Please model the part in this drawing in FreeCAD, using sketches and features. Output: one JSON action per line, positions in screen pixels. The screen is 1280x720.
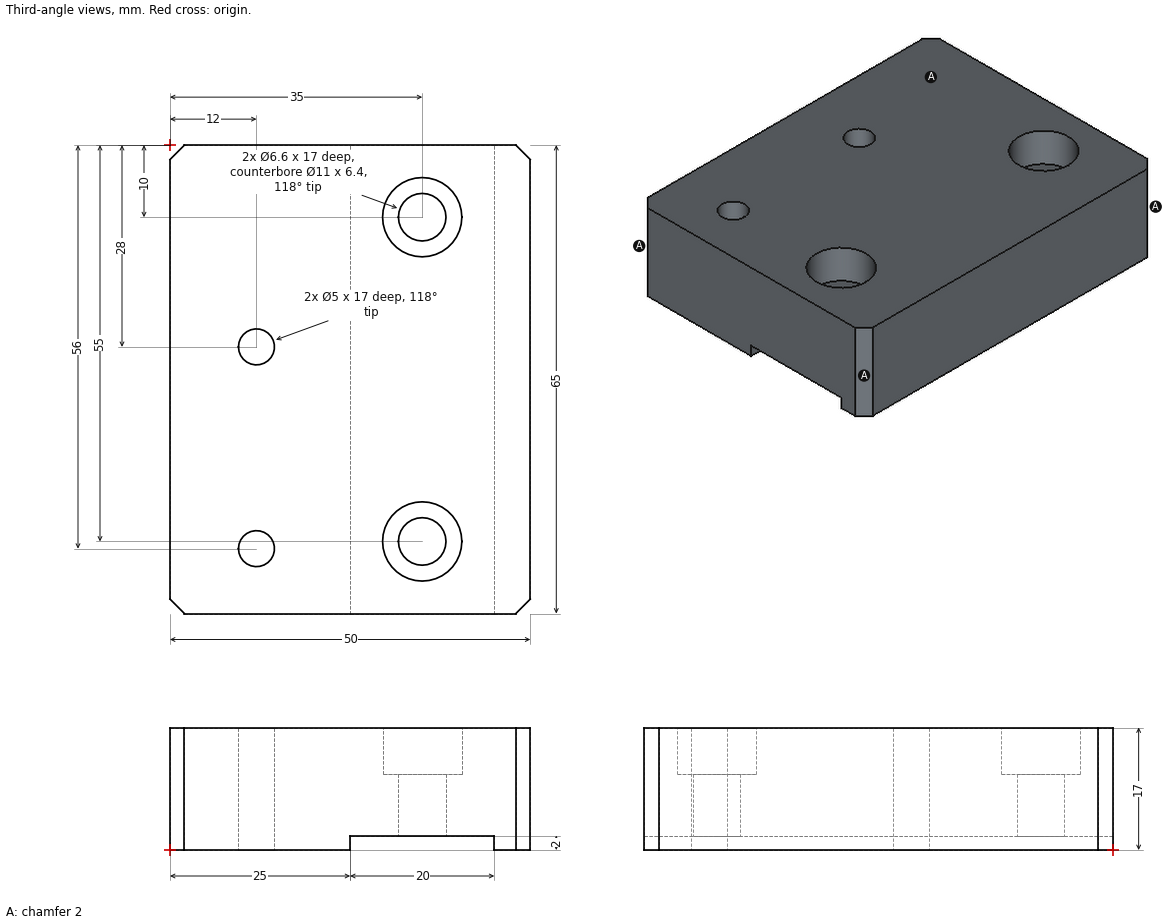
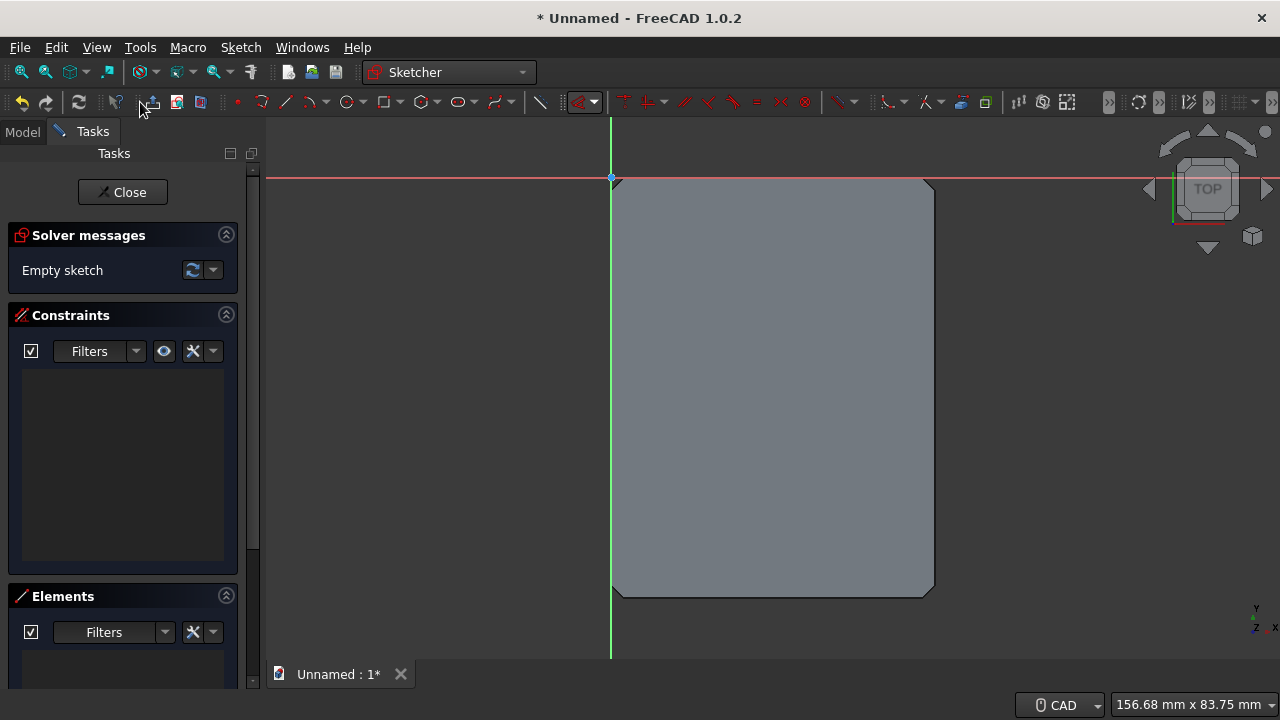
{"action": "left_click", "coordinate": [348, 102]}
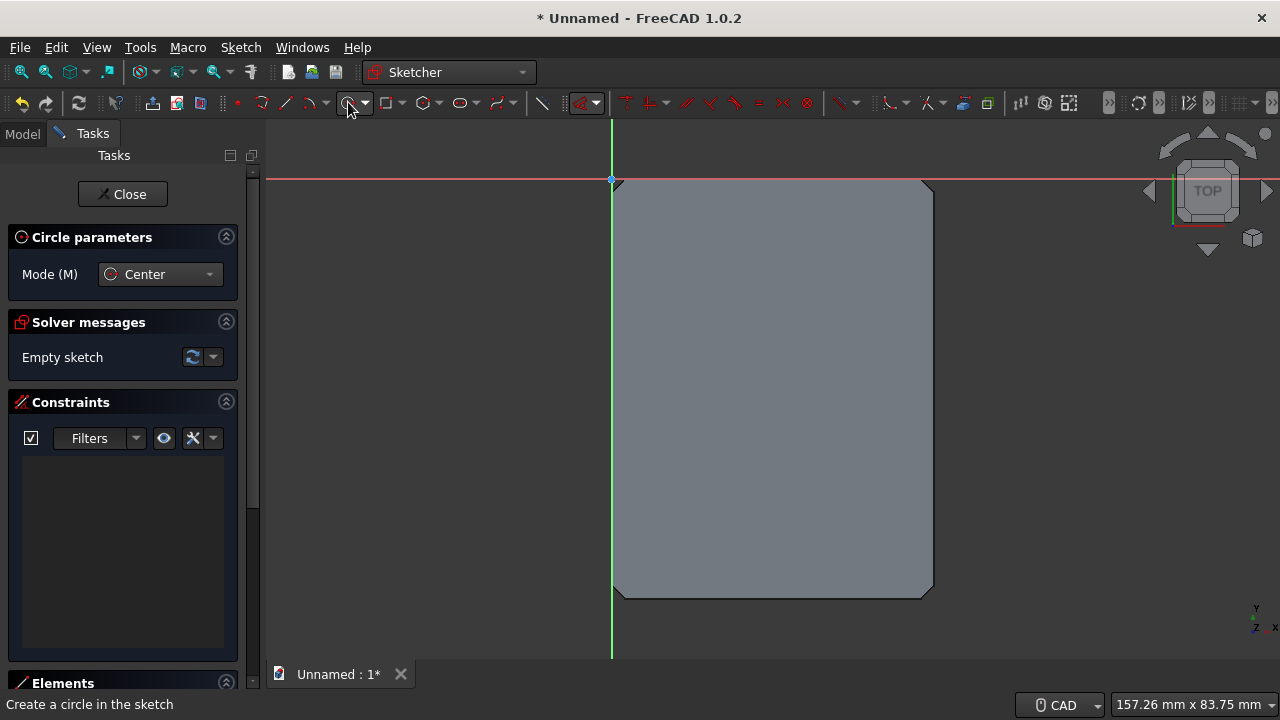
{"action": "scroll", "coordinate": [689, 360], "scroll_direction": "up", "scroll_amount": 2}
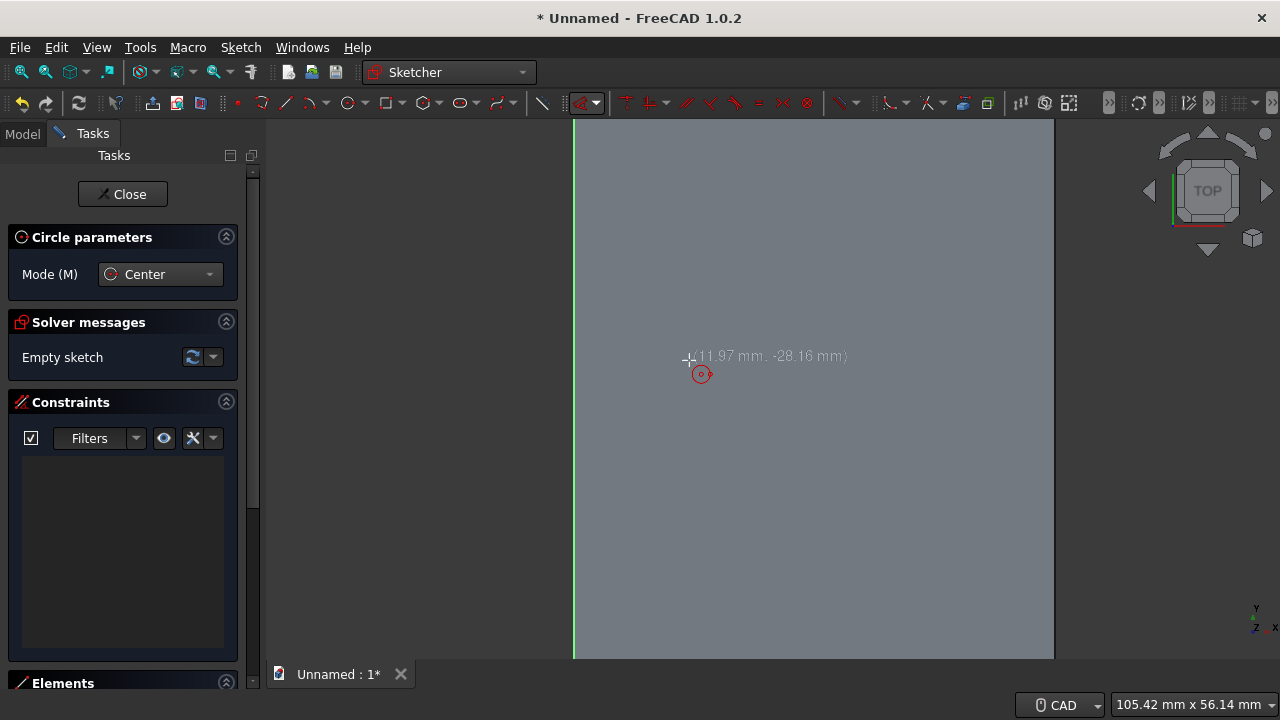
{"action": "left_click", "coordinate": [689, 360]}
{"action": "mouse_move", "coordinate": [706, 343]}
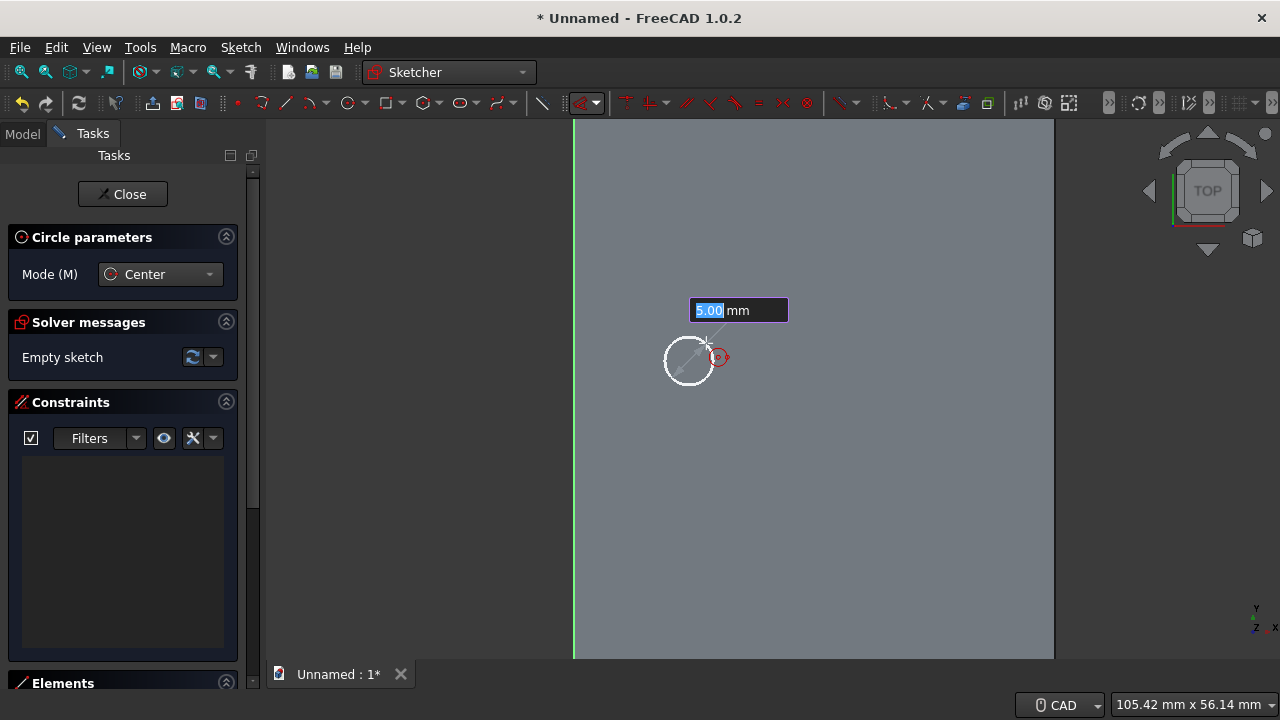
{"action": "type", "text": "5"}
{"action": "key", "text": "Return"}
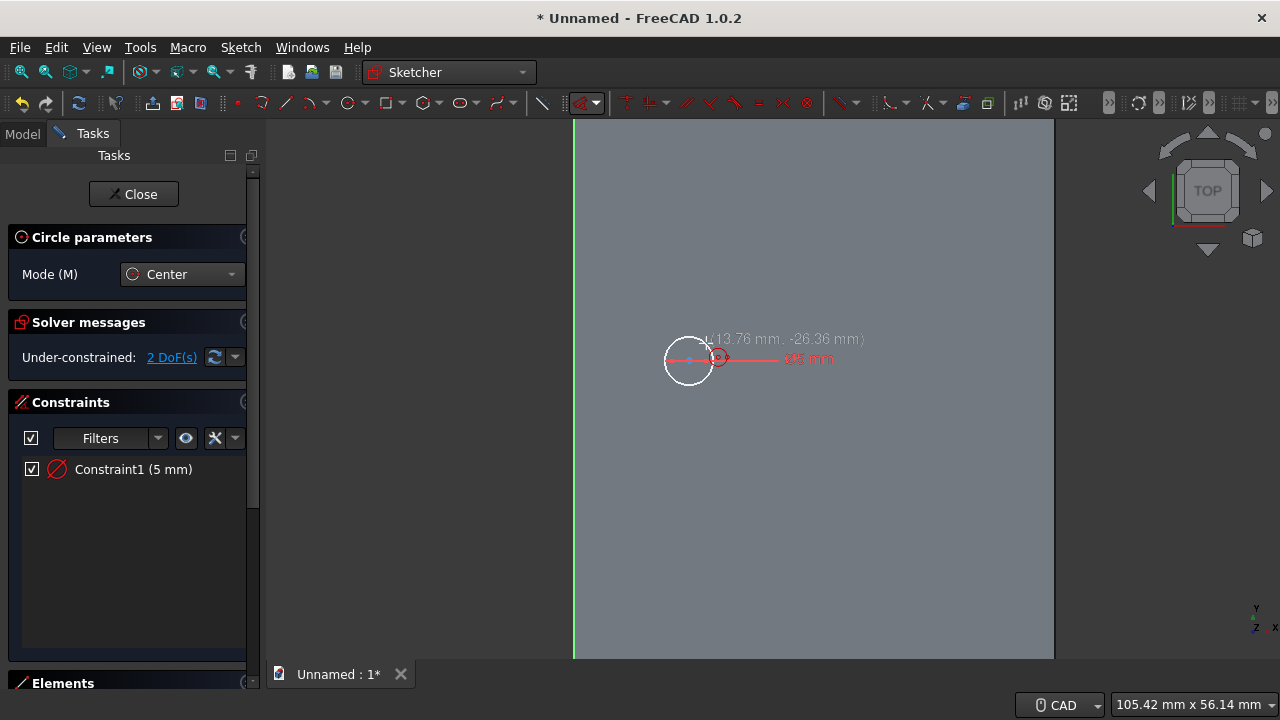
{"action": "left_click", "coordinate": [689, 629]}
{"action": "mouse_move", "coordinate": [706, 612]}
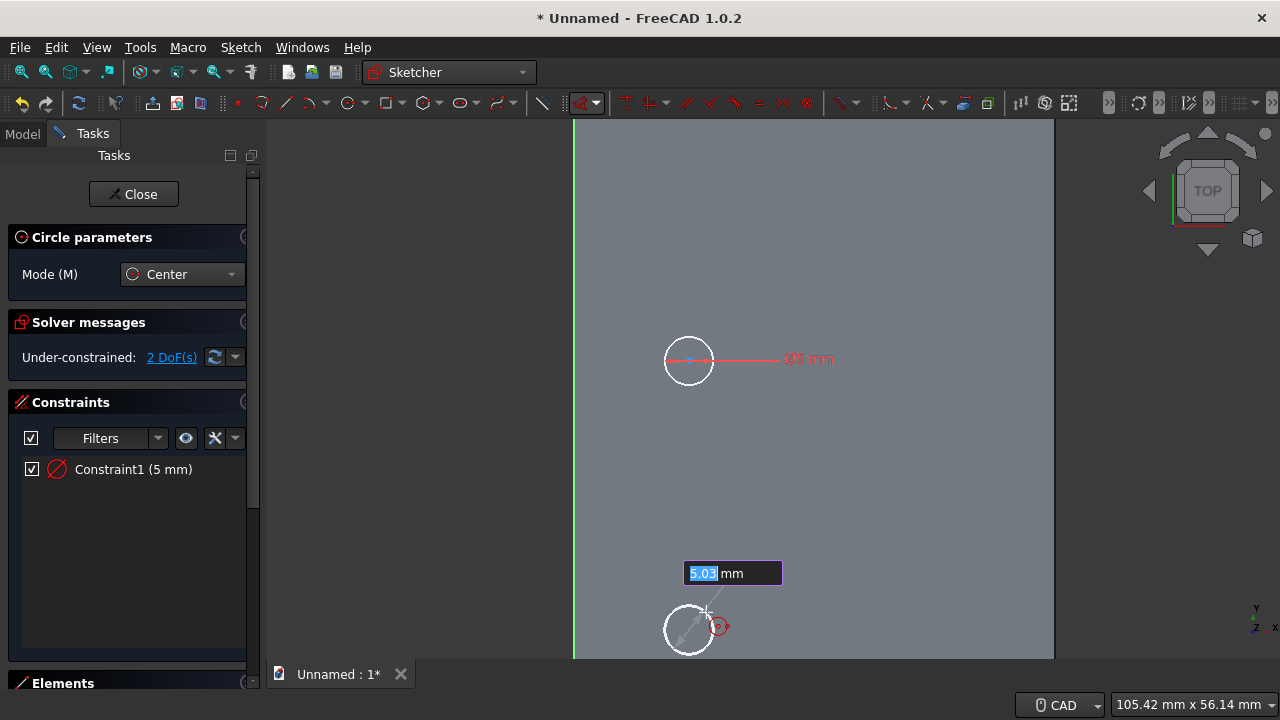
{"action": "type", "text": "5"}
{"action": "key", "text": "Return"}
{"action": "key", "text": "Escape"}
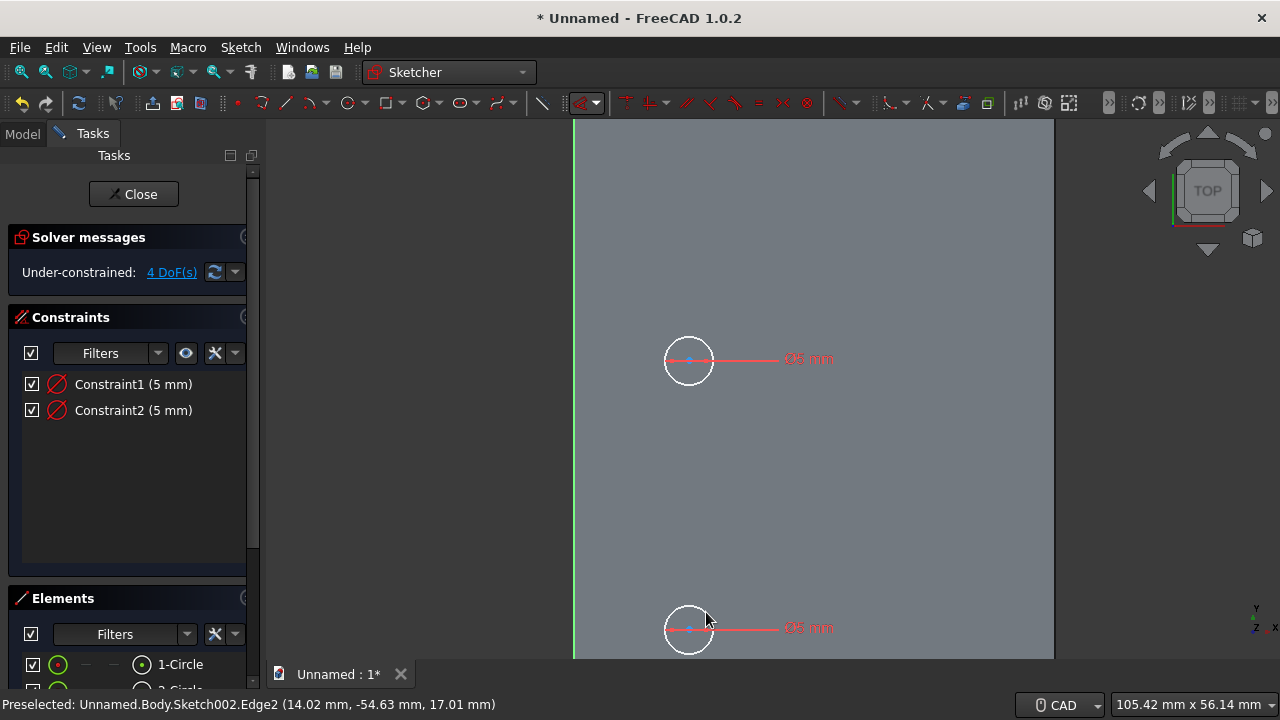
{"action": "left_click", "coordinate": [689, 361]}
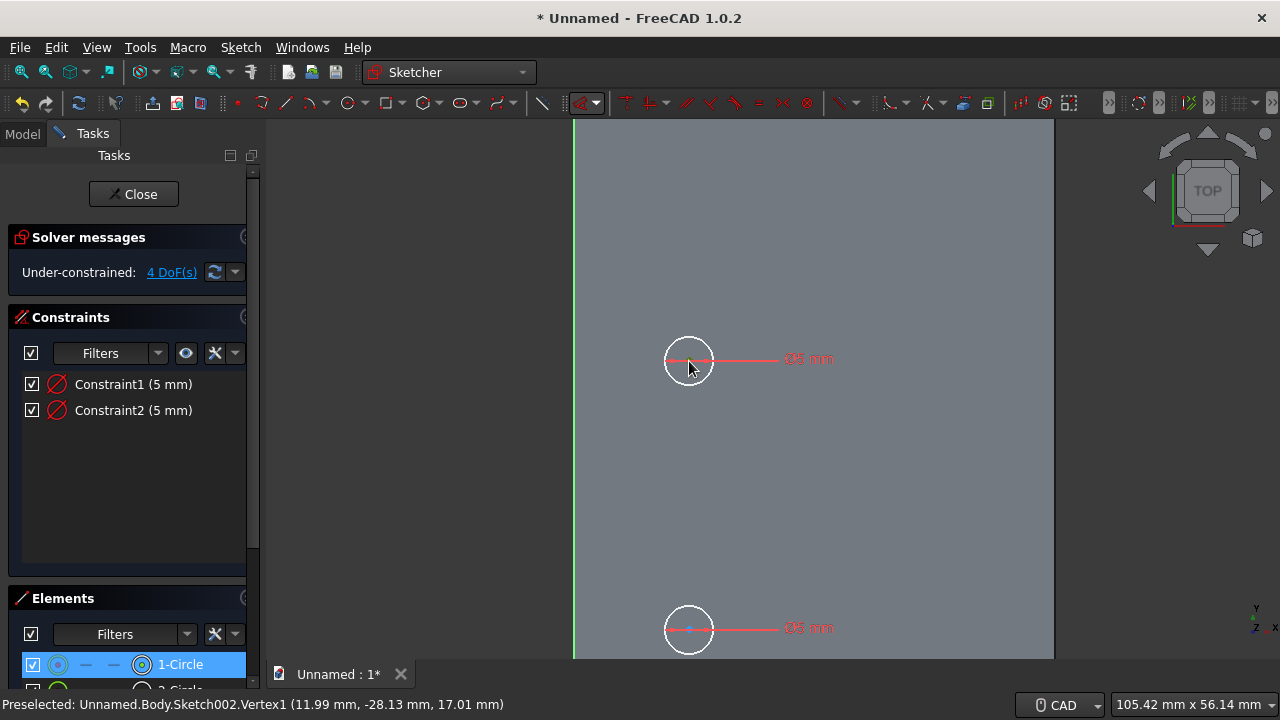
{"action": "left_click", "coordinate": [598, 104]}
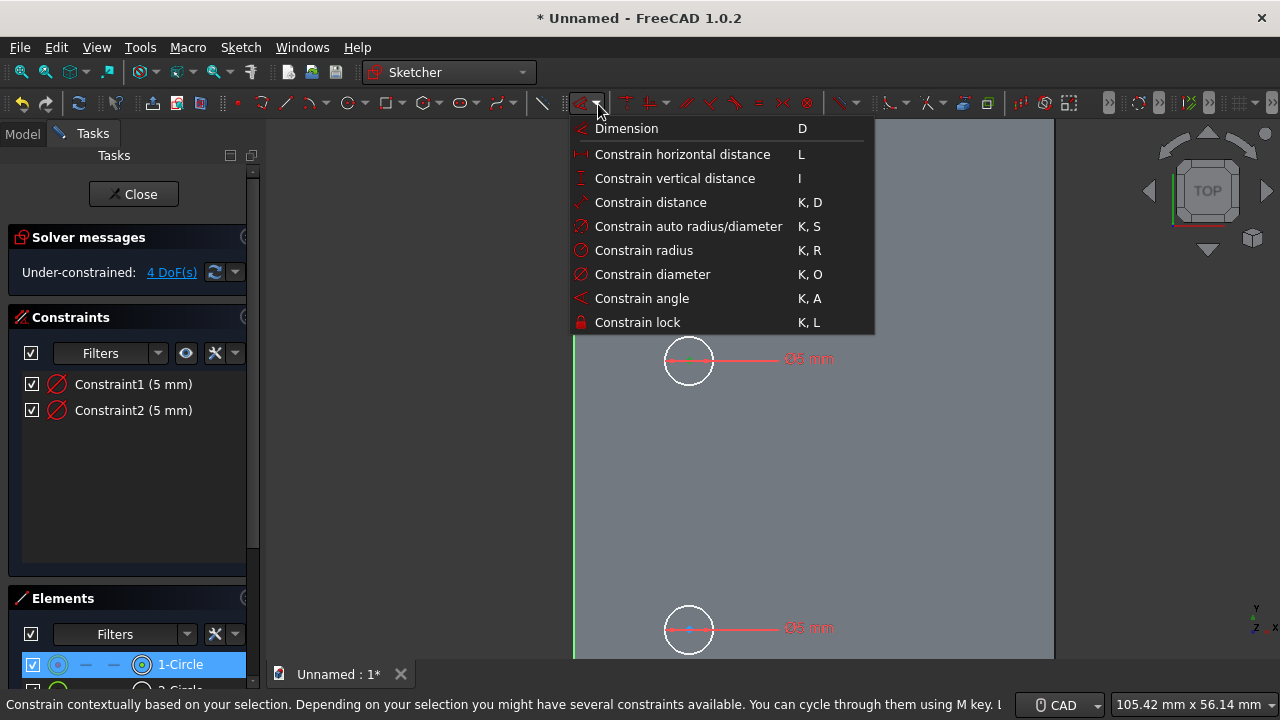
{"action": "left_click", "coordinate": [722, 154]}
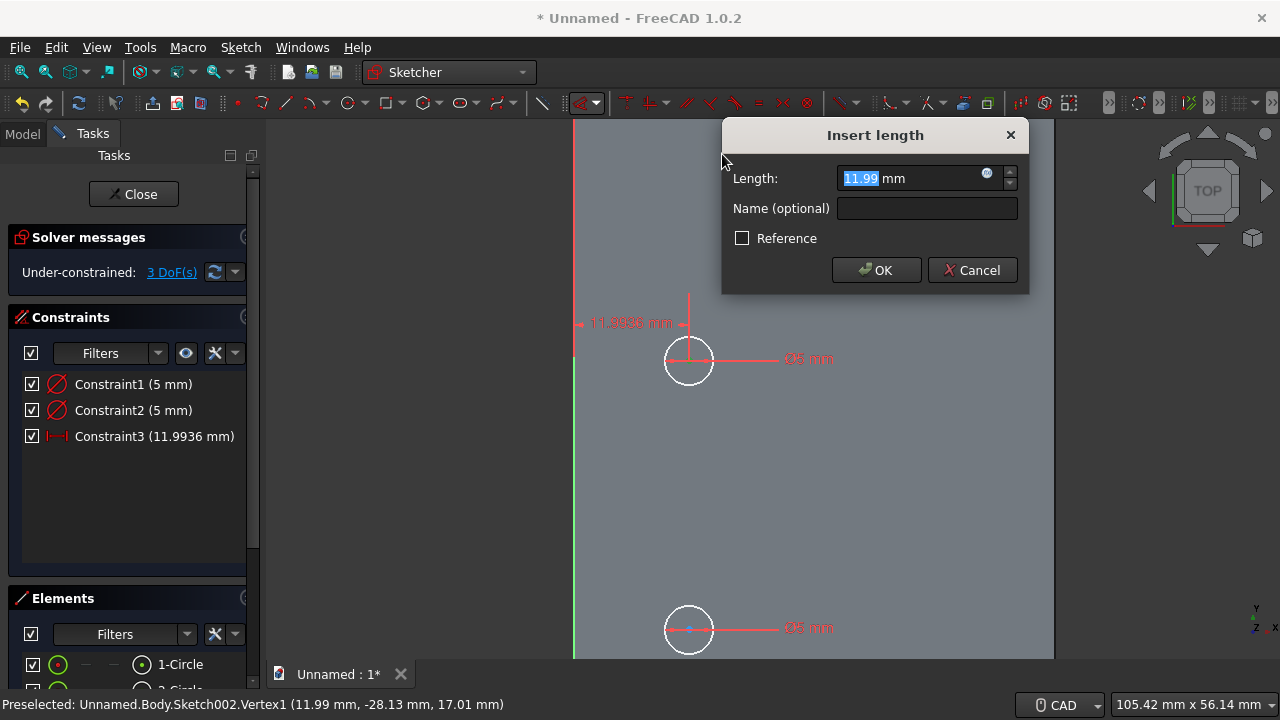
{"action": "type", "text": "12"}
{"action": "key", "text": "Return"}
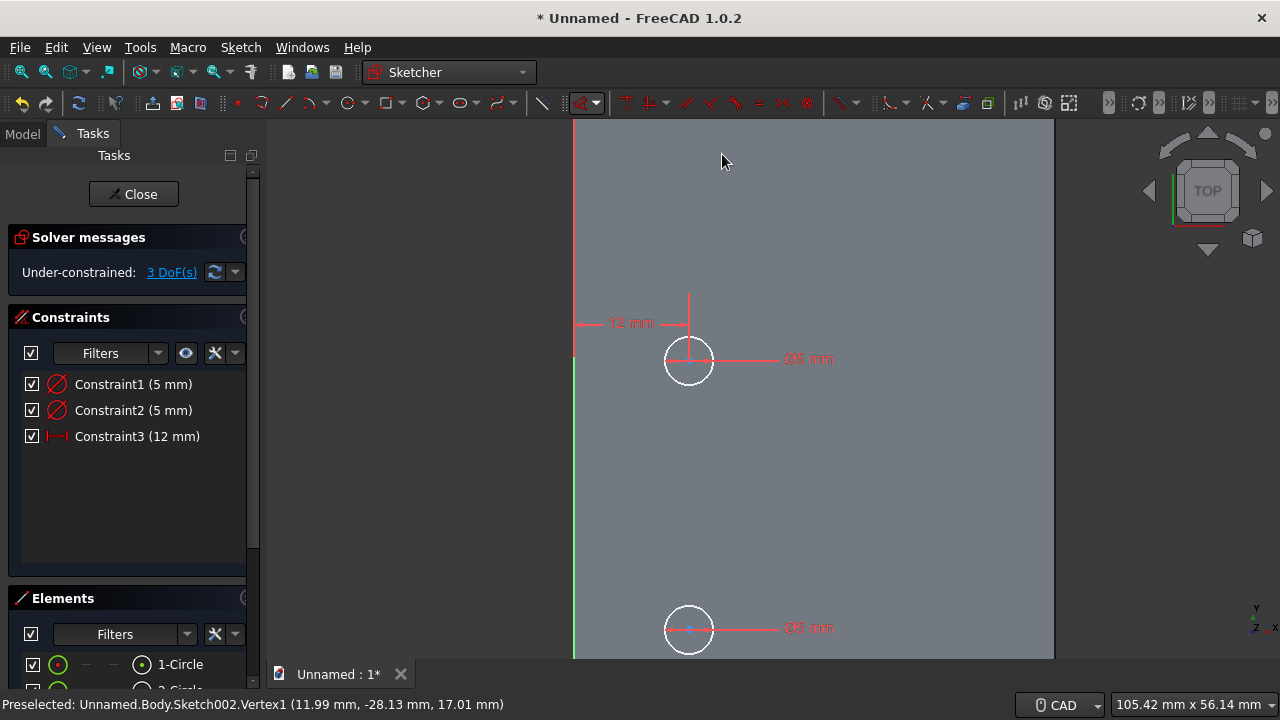
{"action": "left_click", "coordinate": [689, 361]}